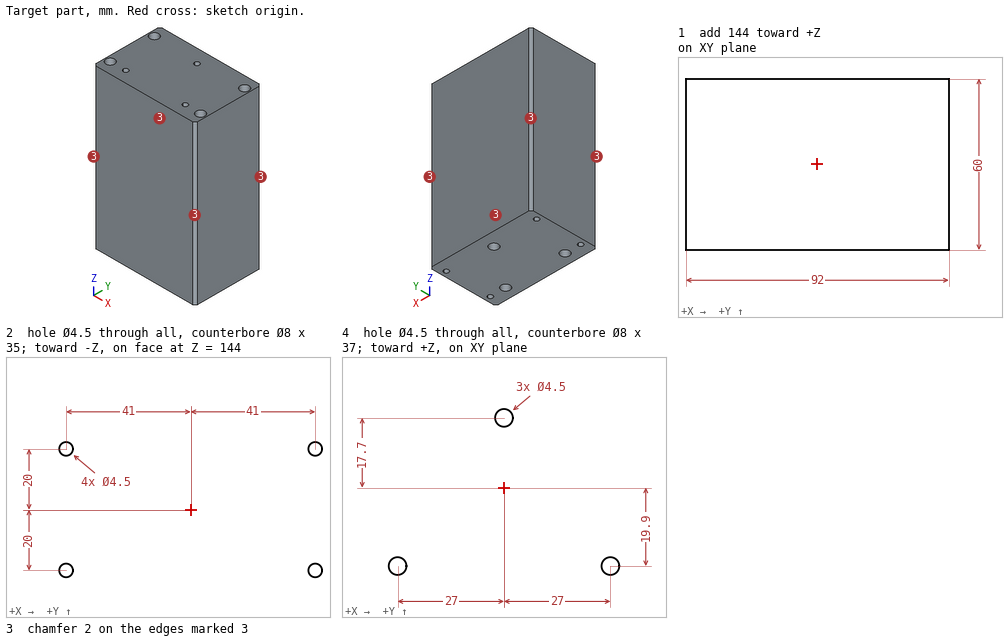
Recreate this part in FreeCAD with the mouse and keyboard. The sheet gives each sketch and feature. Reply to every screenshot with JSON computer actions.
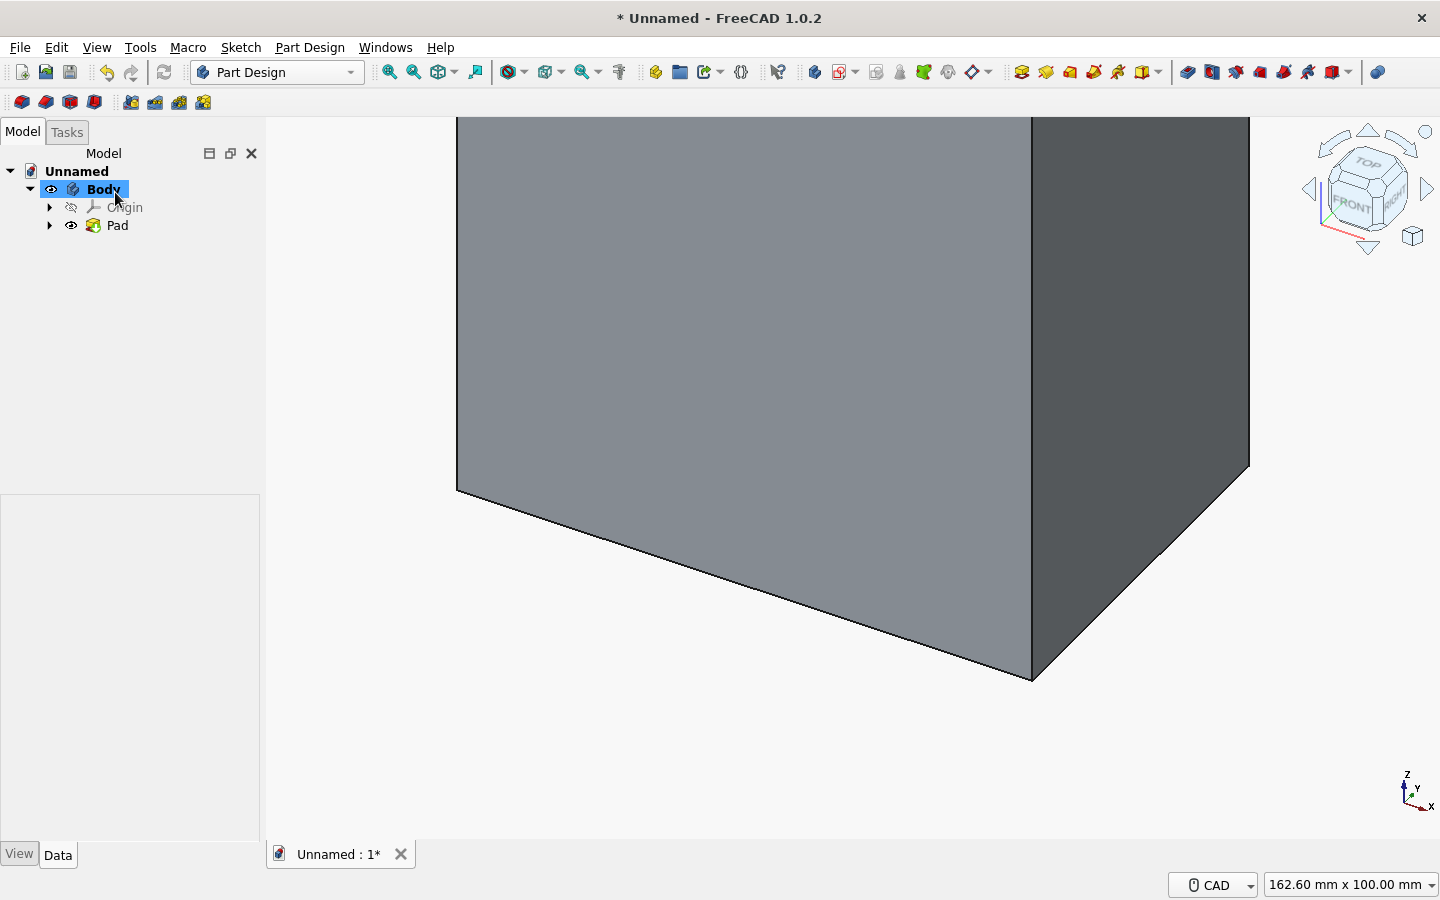
{"action": "left_click", "coordinate": [390, 72]}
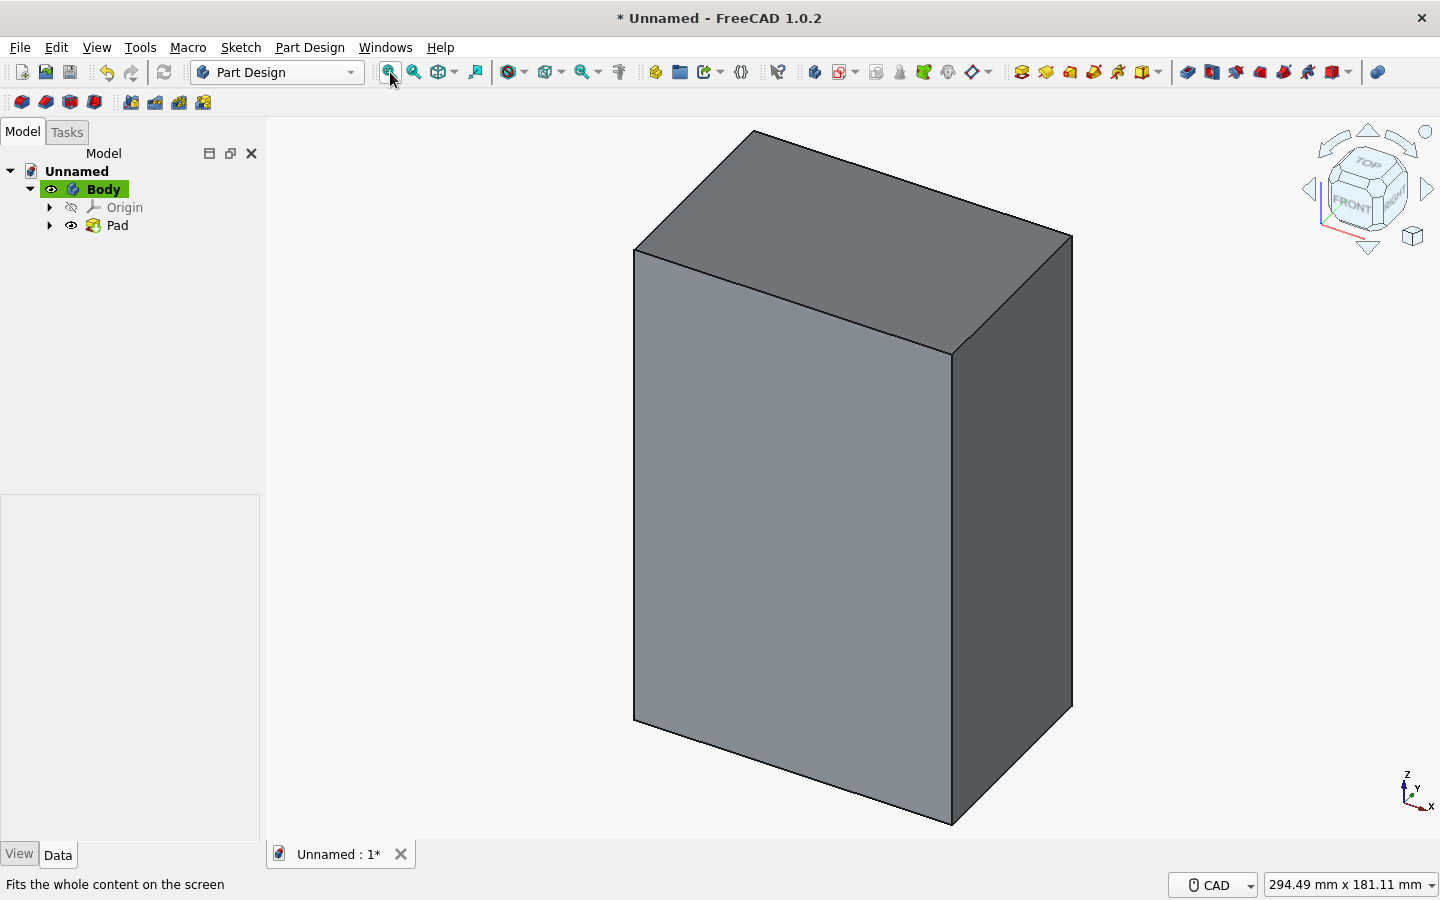
{"action": "left_click", "coordinate": [898, 257]}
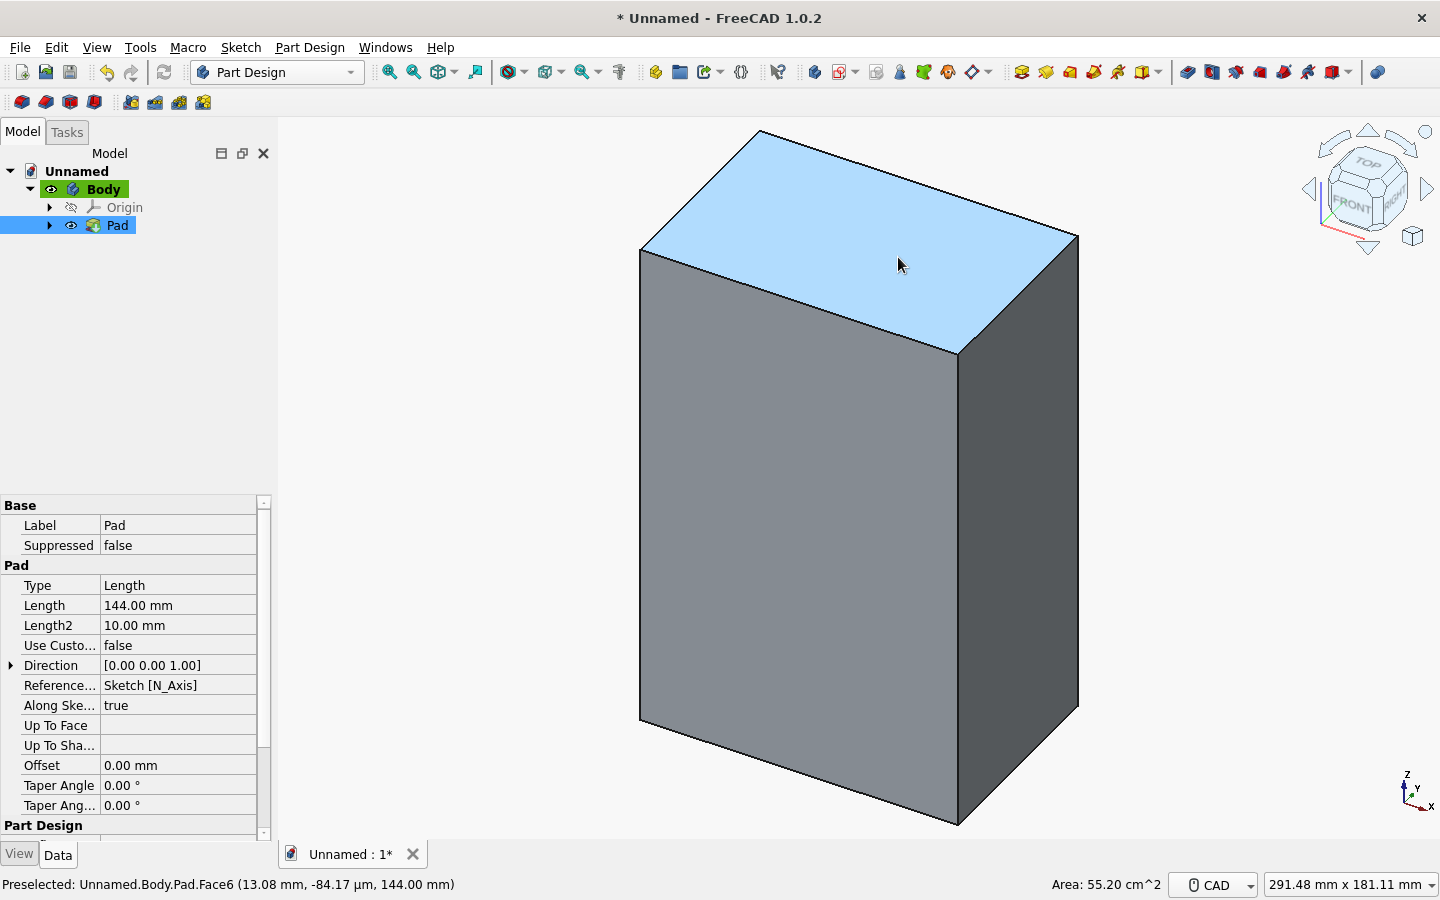
{"action": "left_click", "coordinate": [840, 72]}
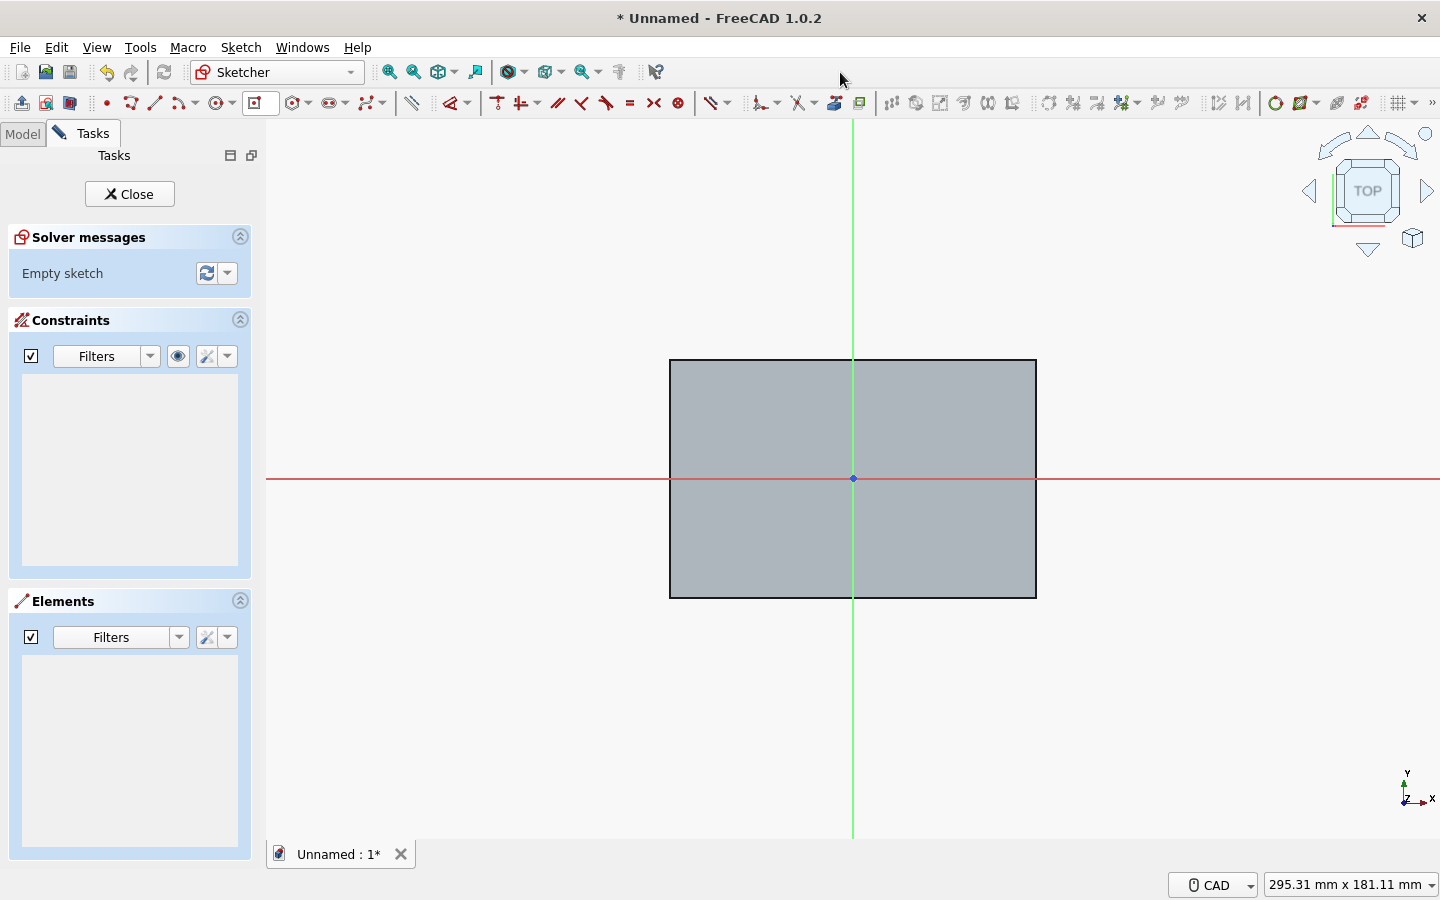
{"action": "scroll", "coordinate": [936, 479], "scroll_direction": "up", "scroll_amount": 3}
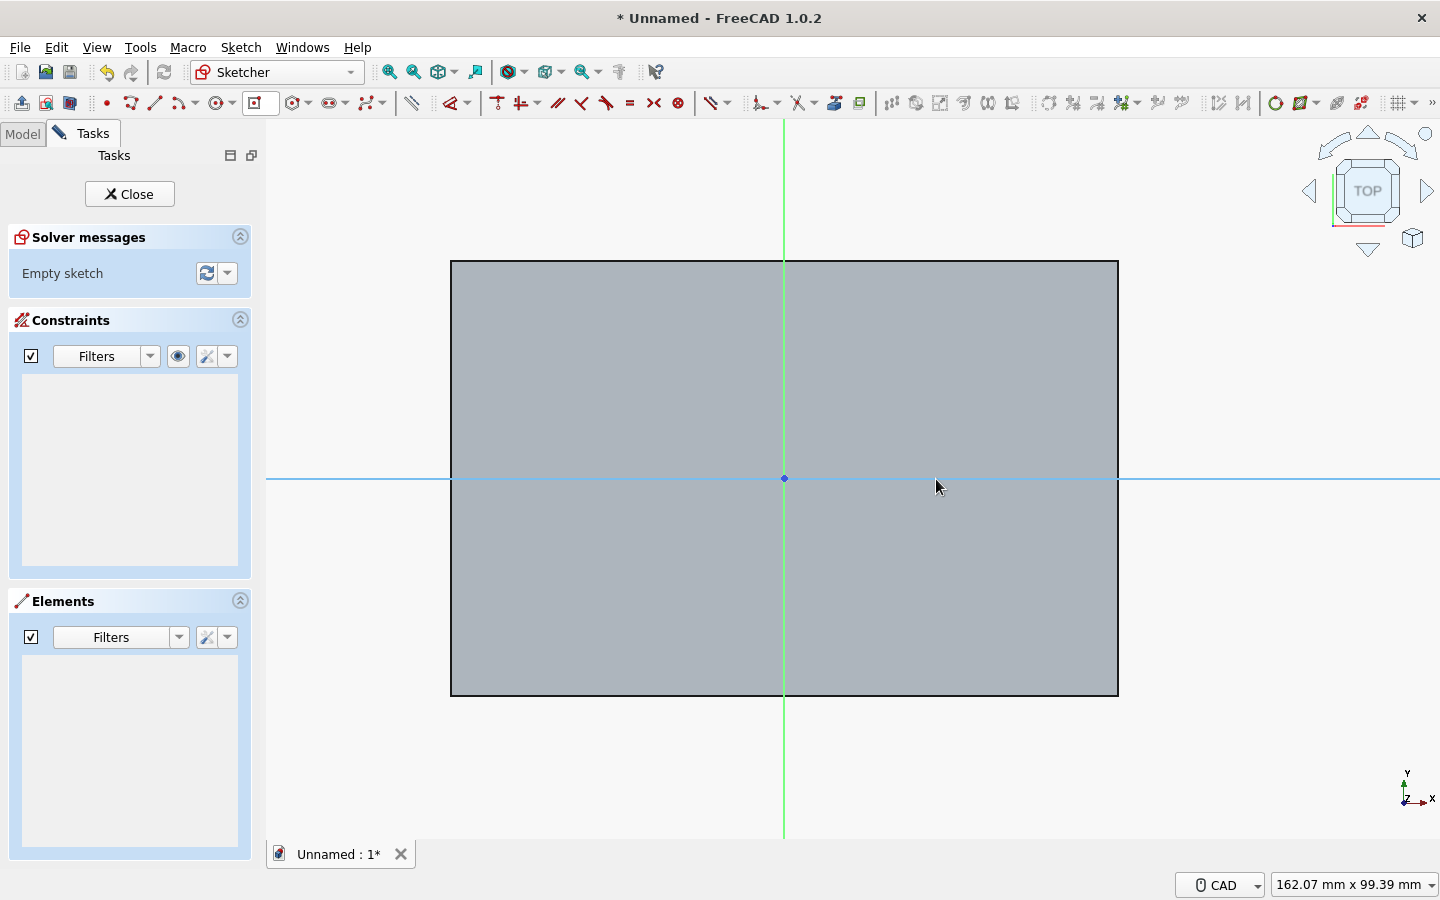
{"action": "left_click", "coordinate": [216, 104]}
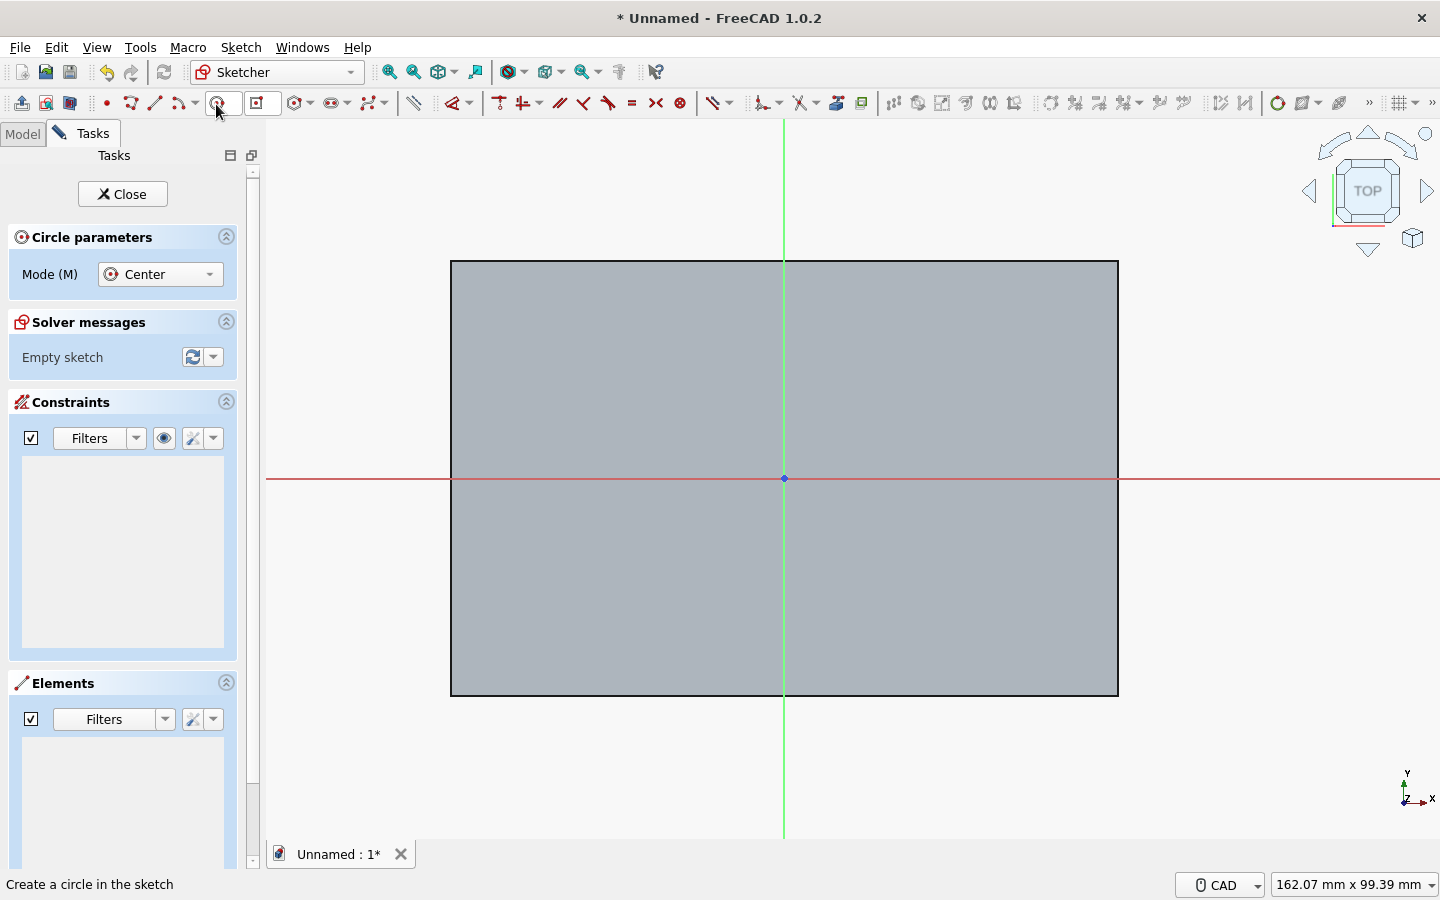
{"action": "scroll", "coordinate": [487, 334], "scroll_direction": "up", "scroll_amount": 2}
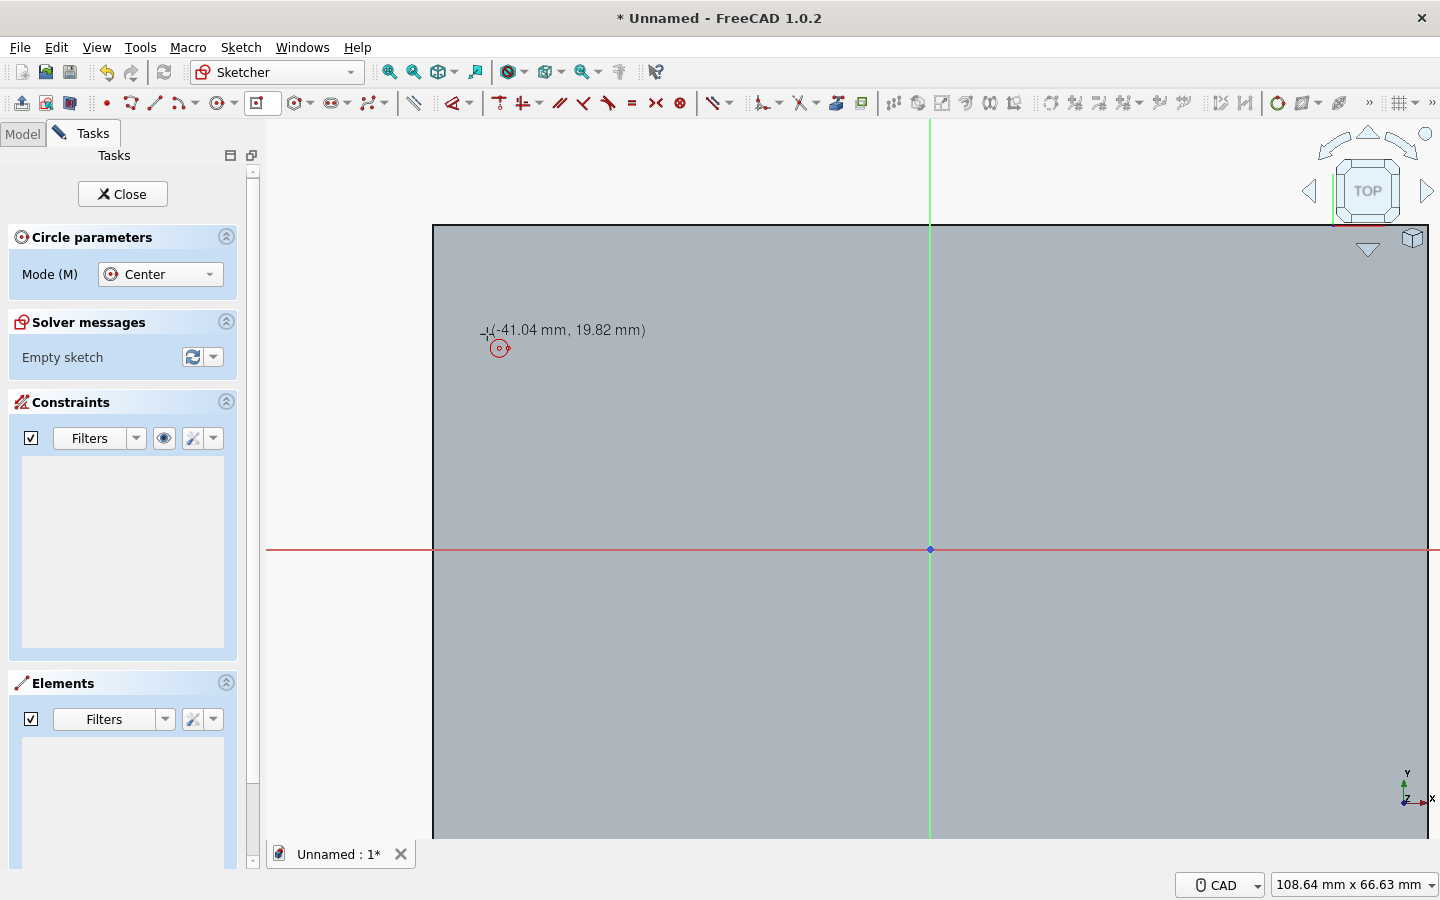
{"action": "left_click", "coordinate": [487, 333]}
{"action": "left_click", "coordinate": [505, 316]}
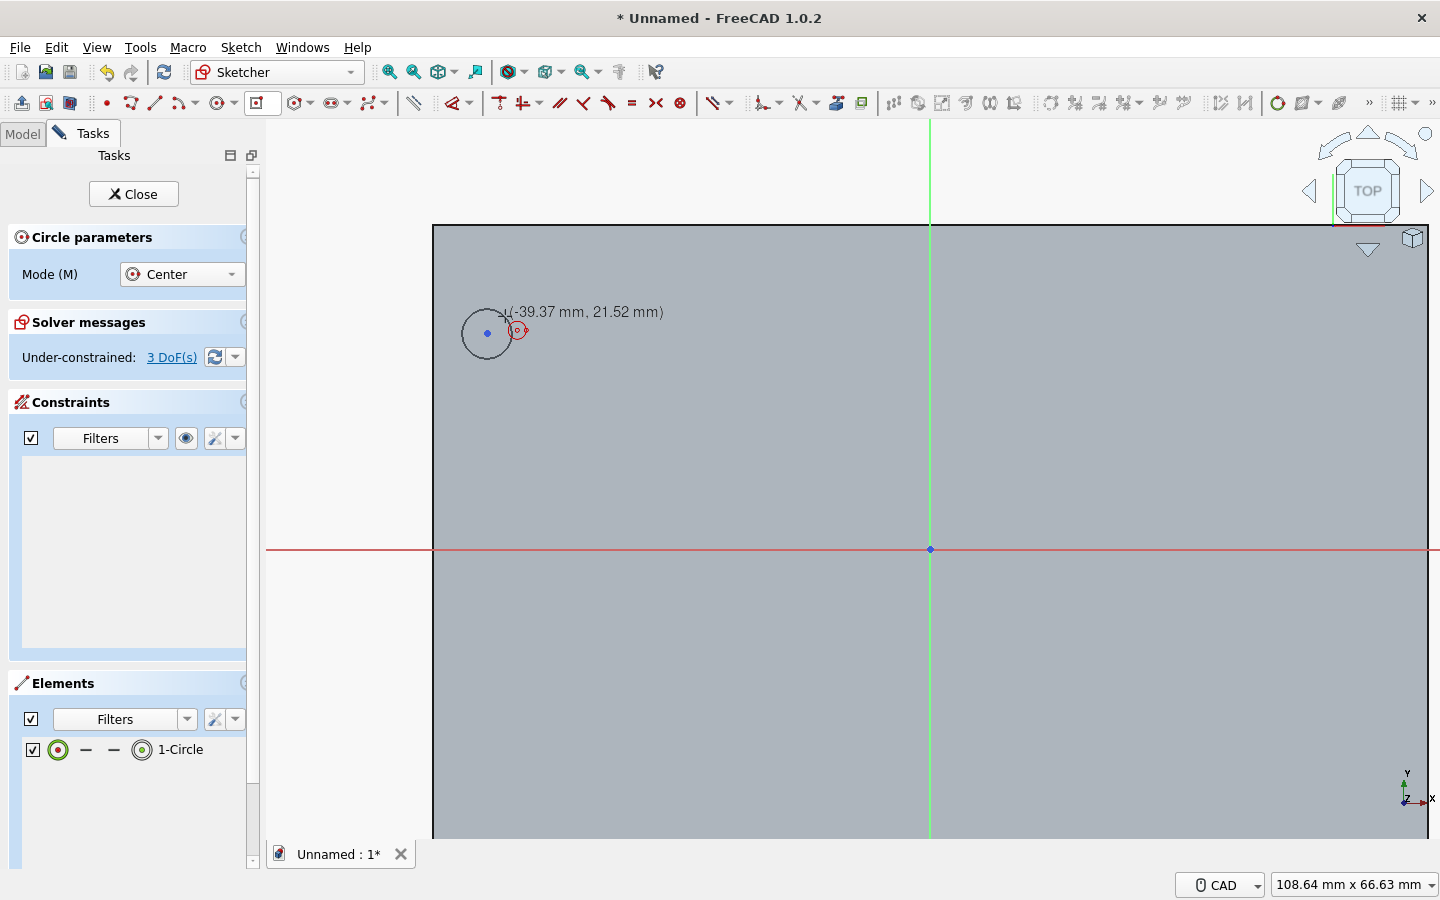
{"action": "left_click", "coordinate": [487, 766]}
{"action": "left_click", "coordinate": [505, 748]}